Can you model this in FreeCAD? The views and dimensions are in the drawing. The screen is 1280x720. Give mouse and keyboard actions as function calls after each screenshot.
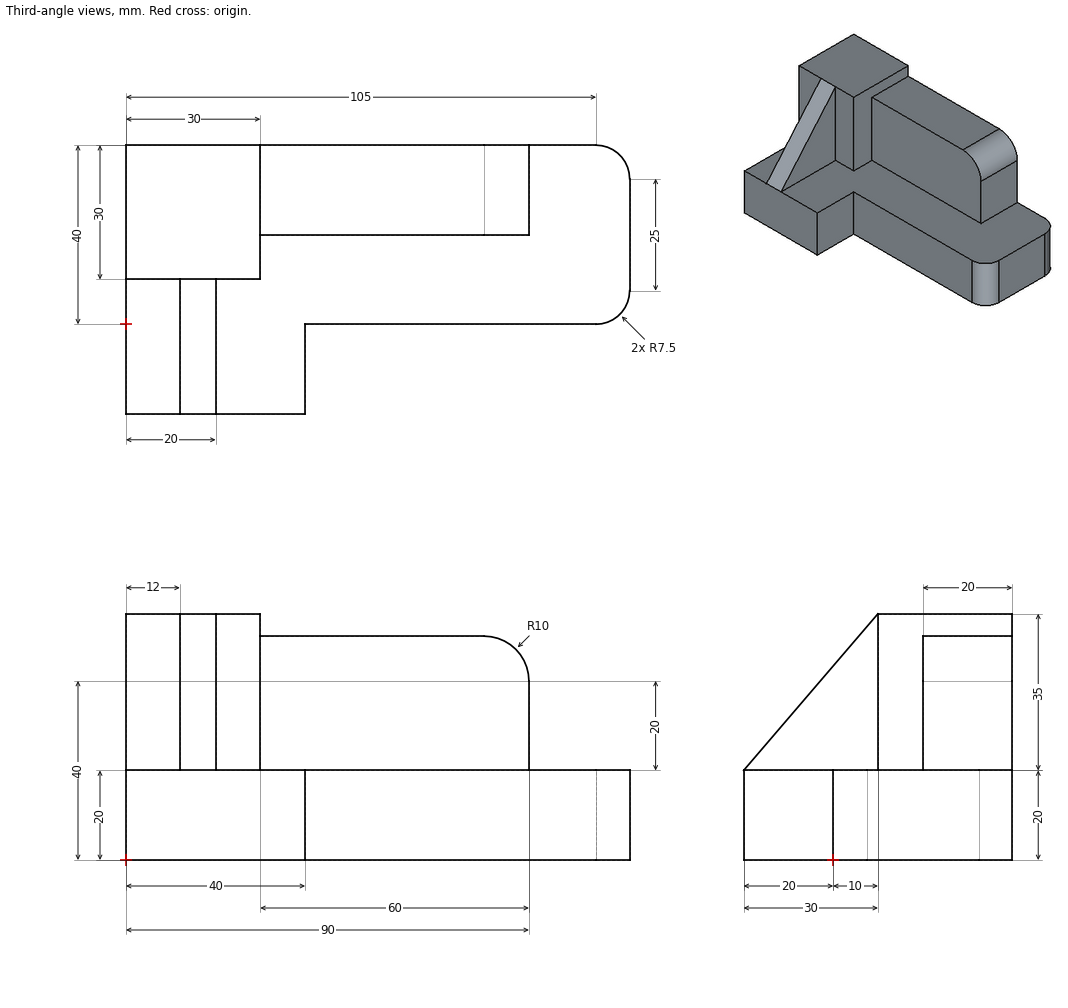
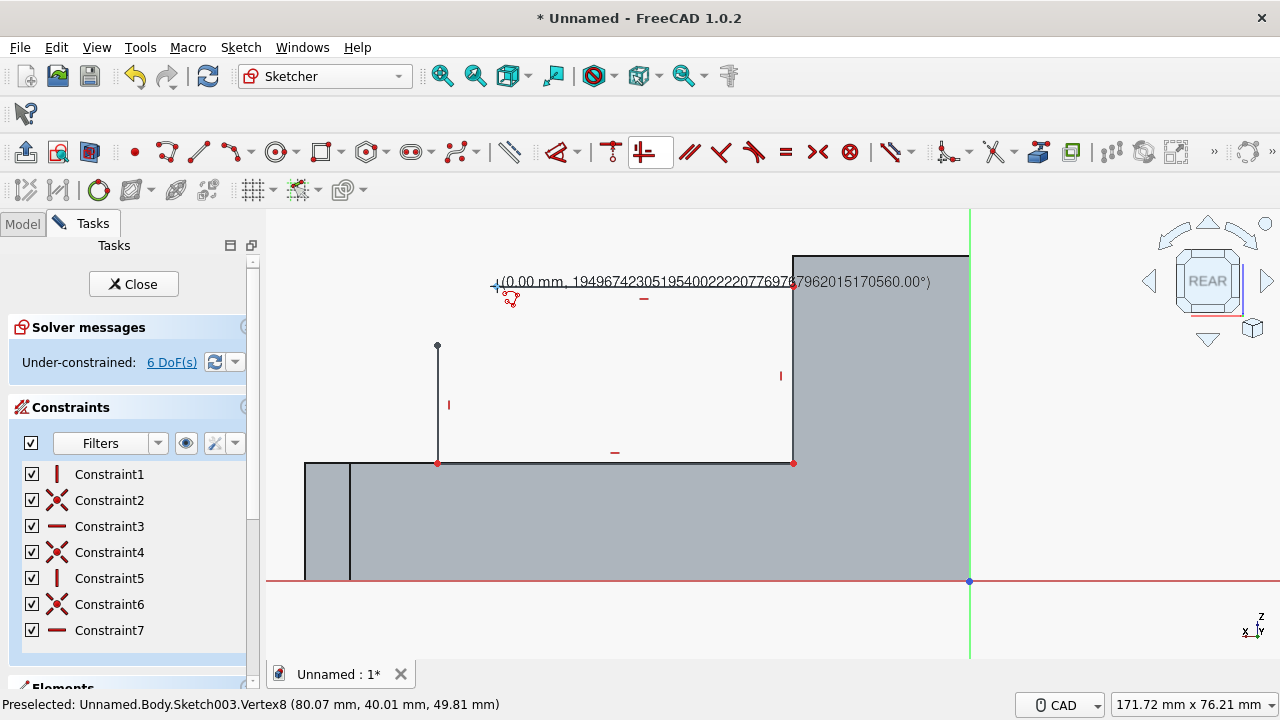
click(232, 152)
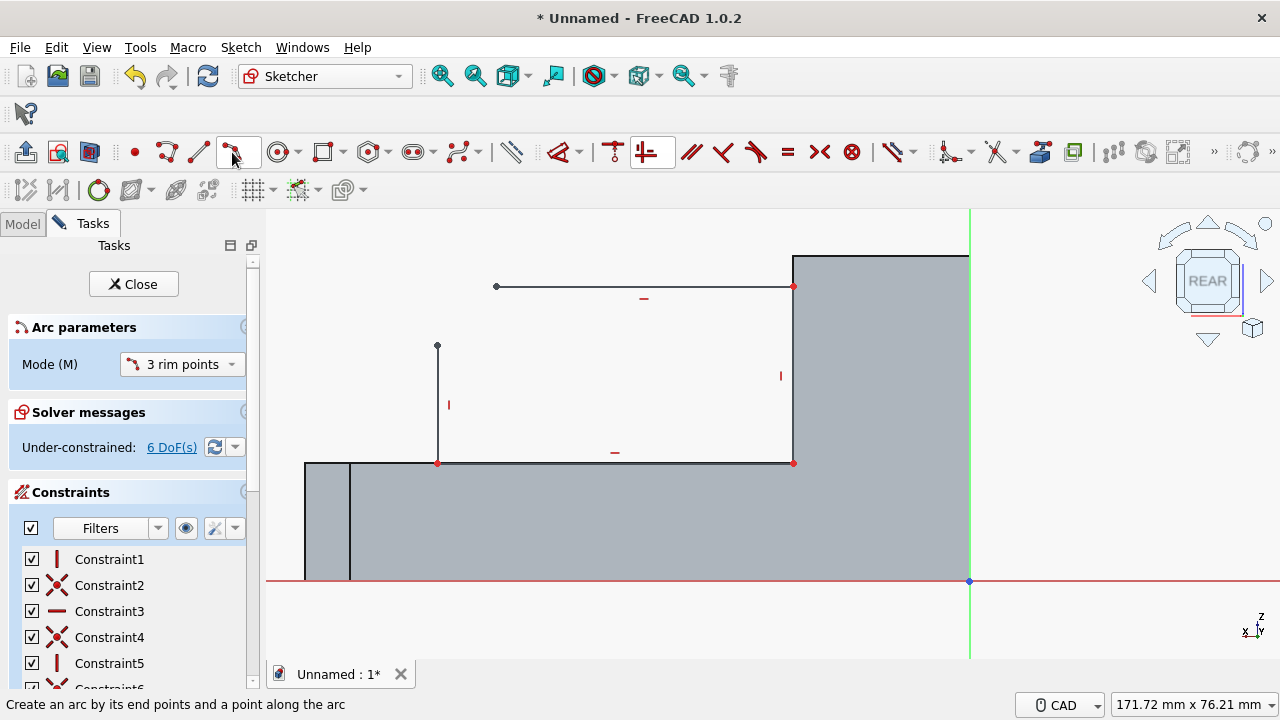
click(497, 287)
click(438, 346)
click(456, 303)
key(Escape)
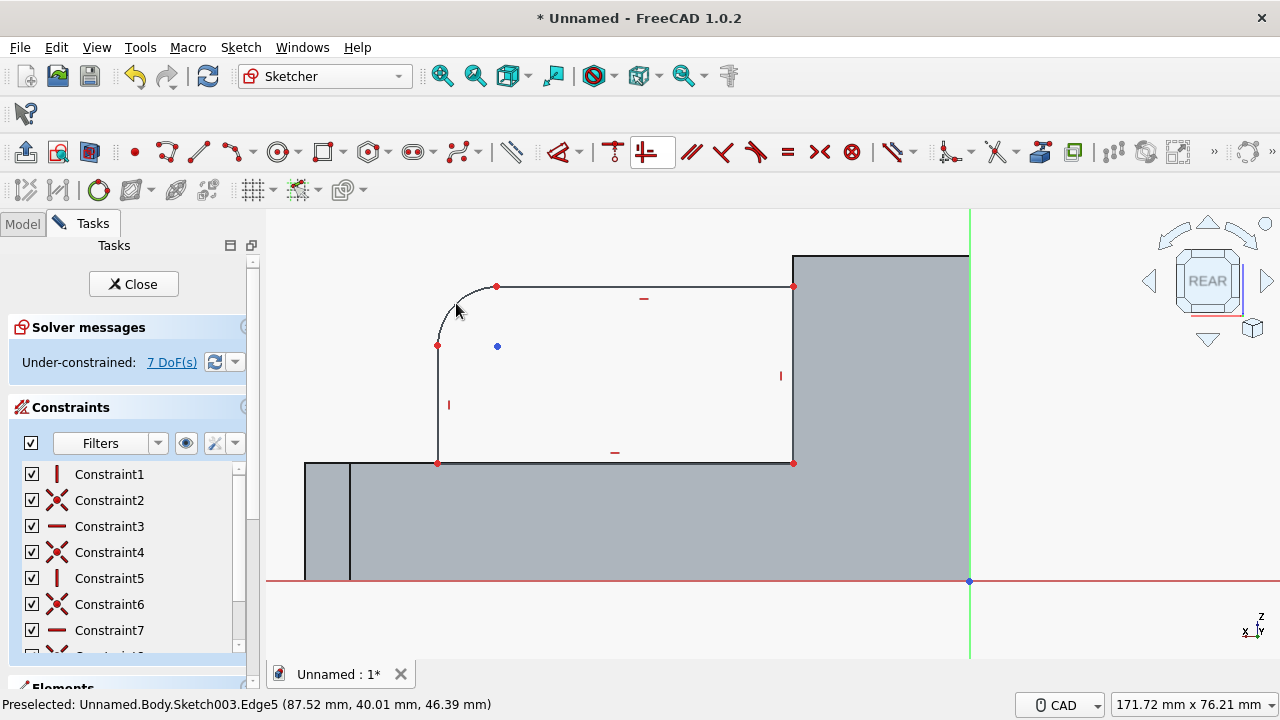
click(438, 381)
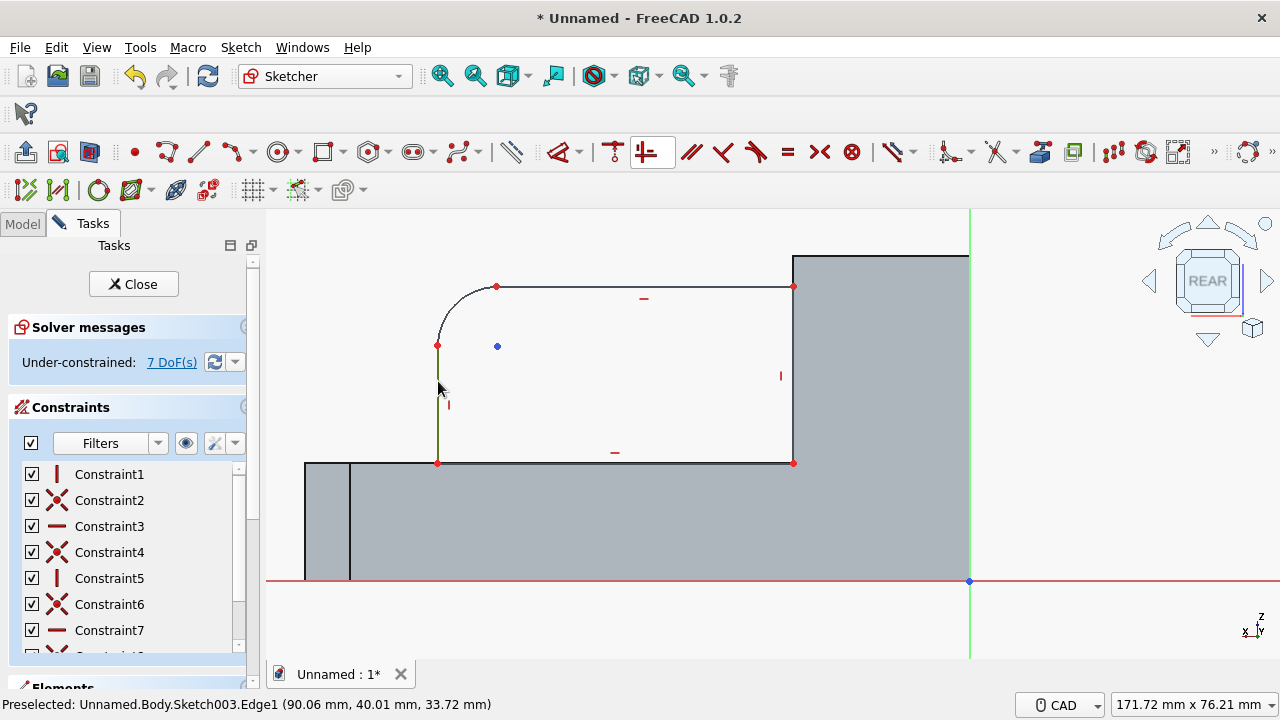
click(470, 294)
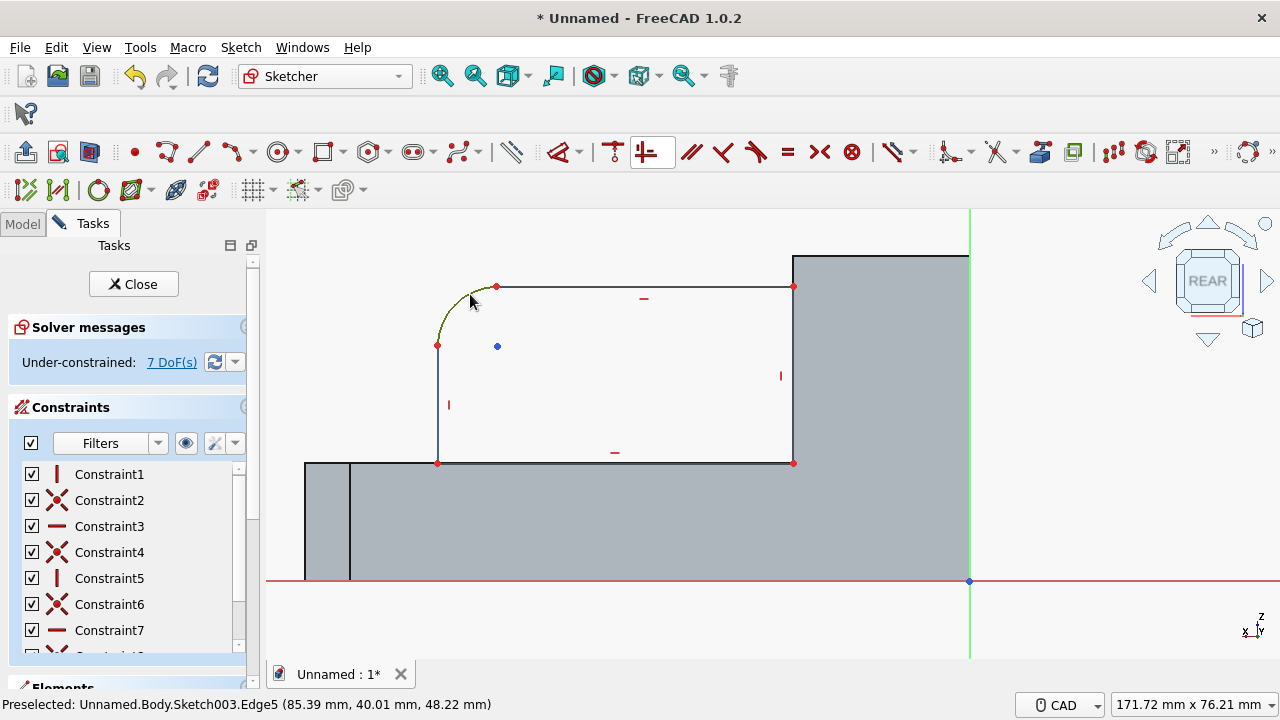
key(t)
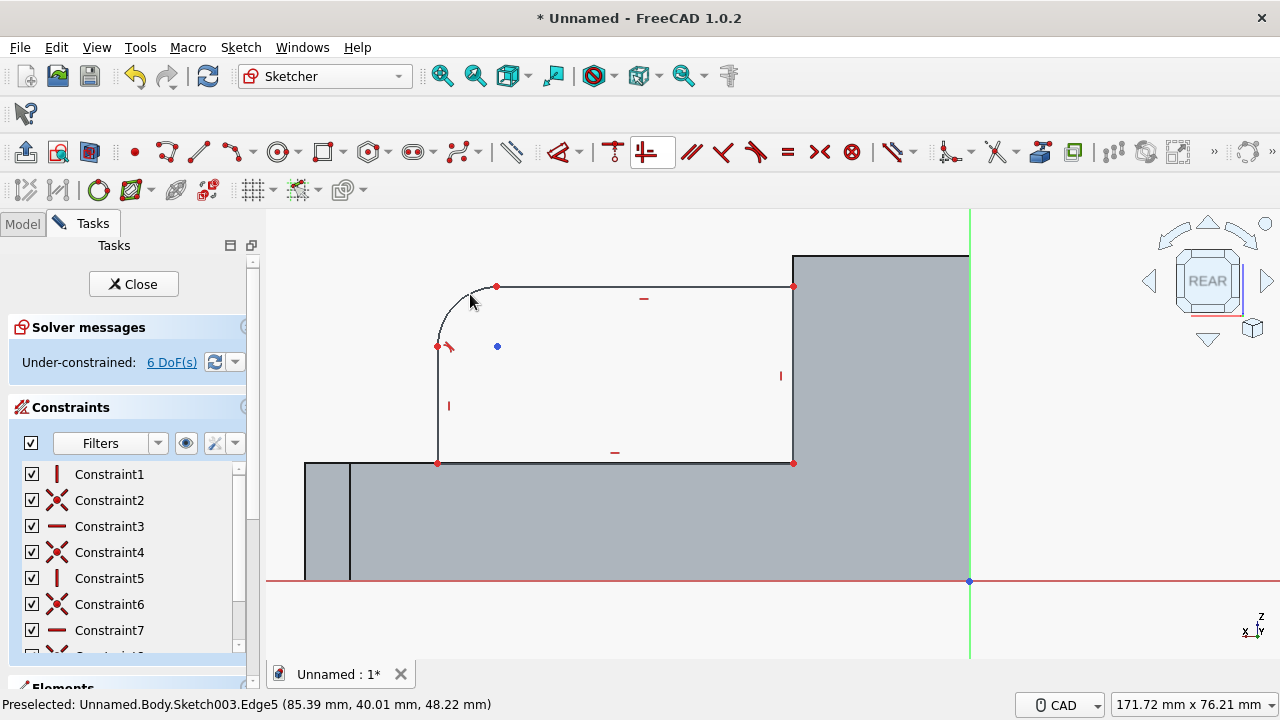
click(704, 287)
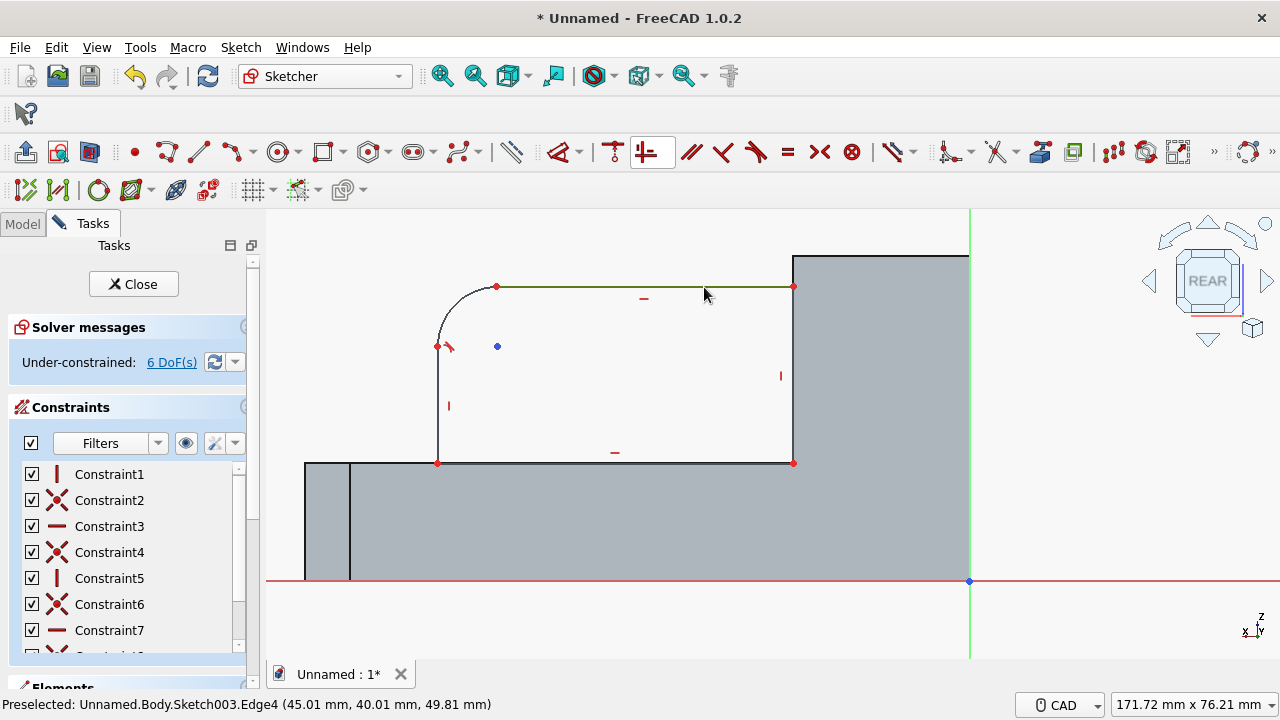
click(470, 294)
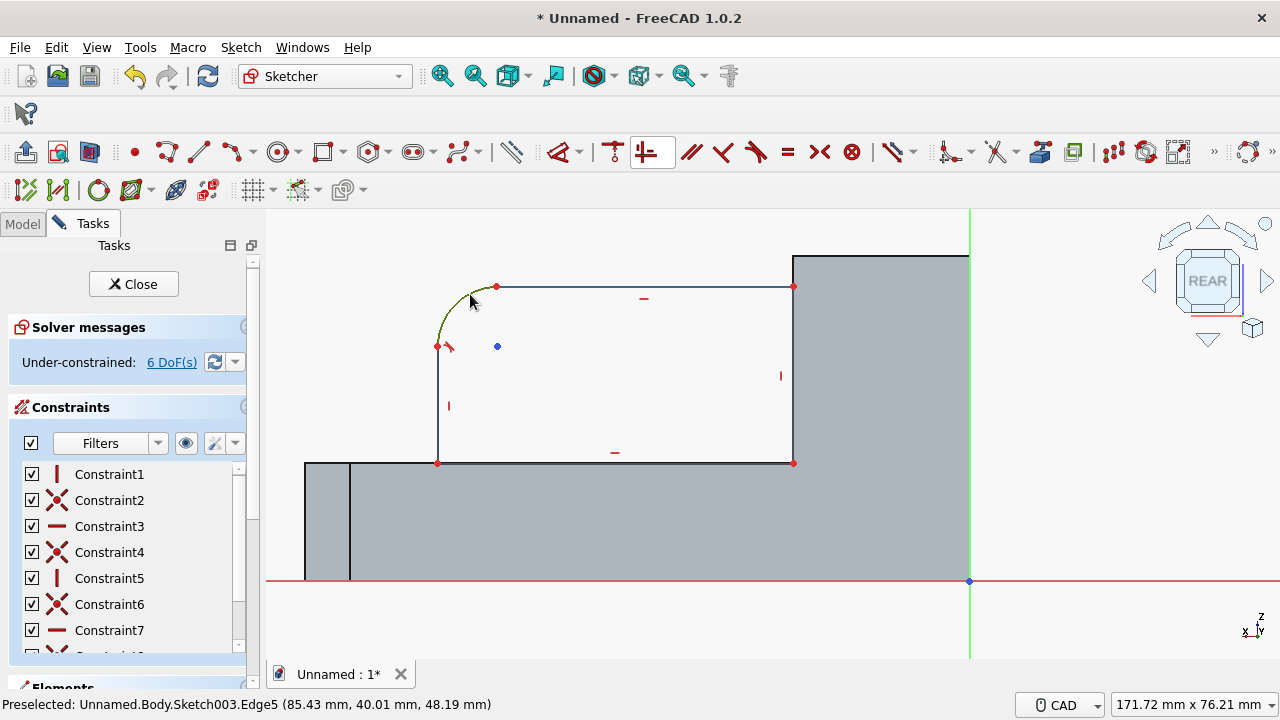
key(t)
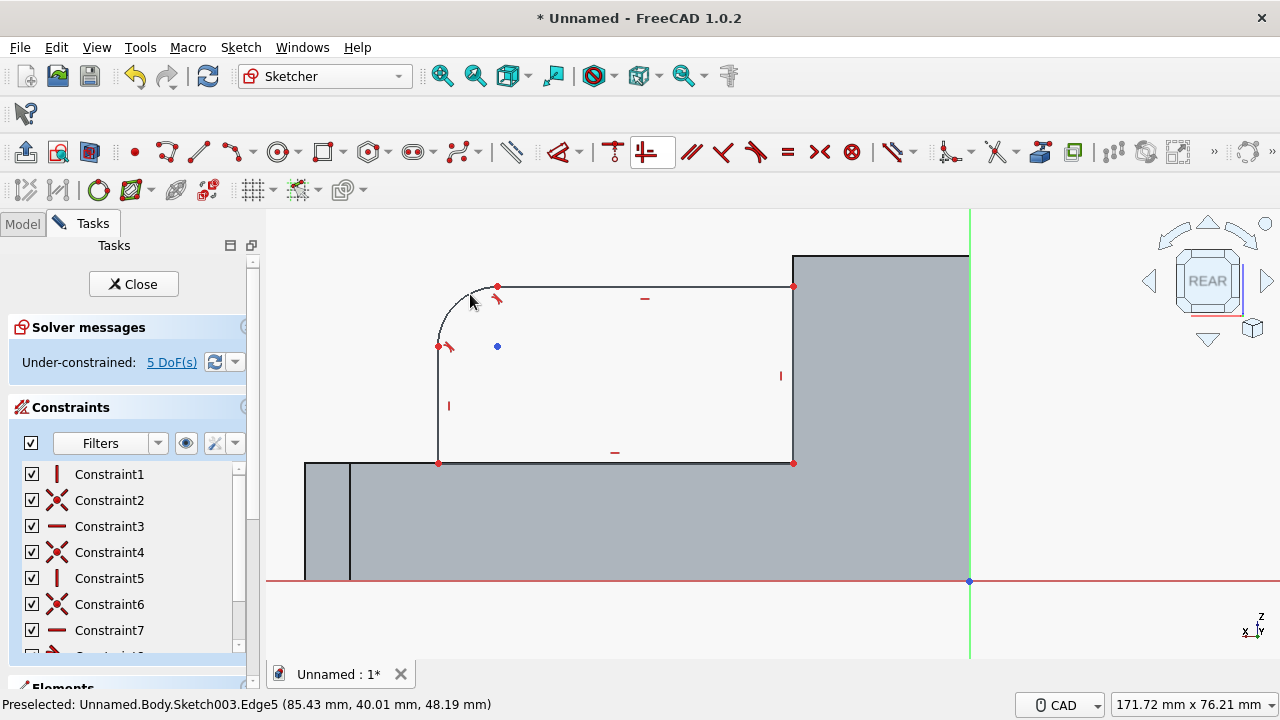
key(d)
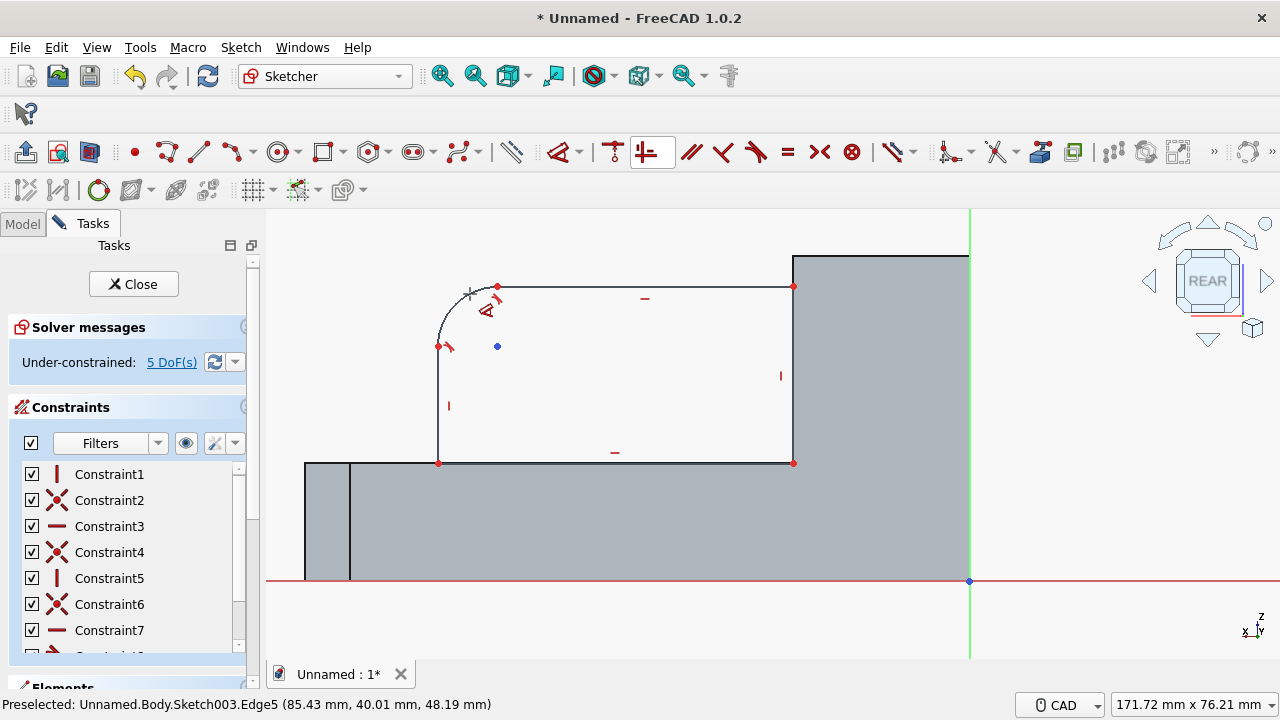
click(471, 294)
click(457, 265)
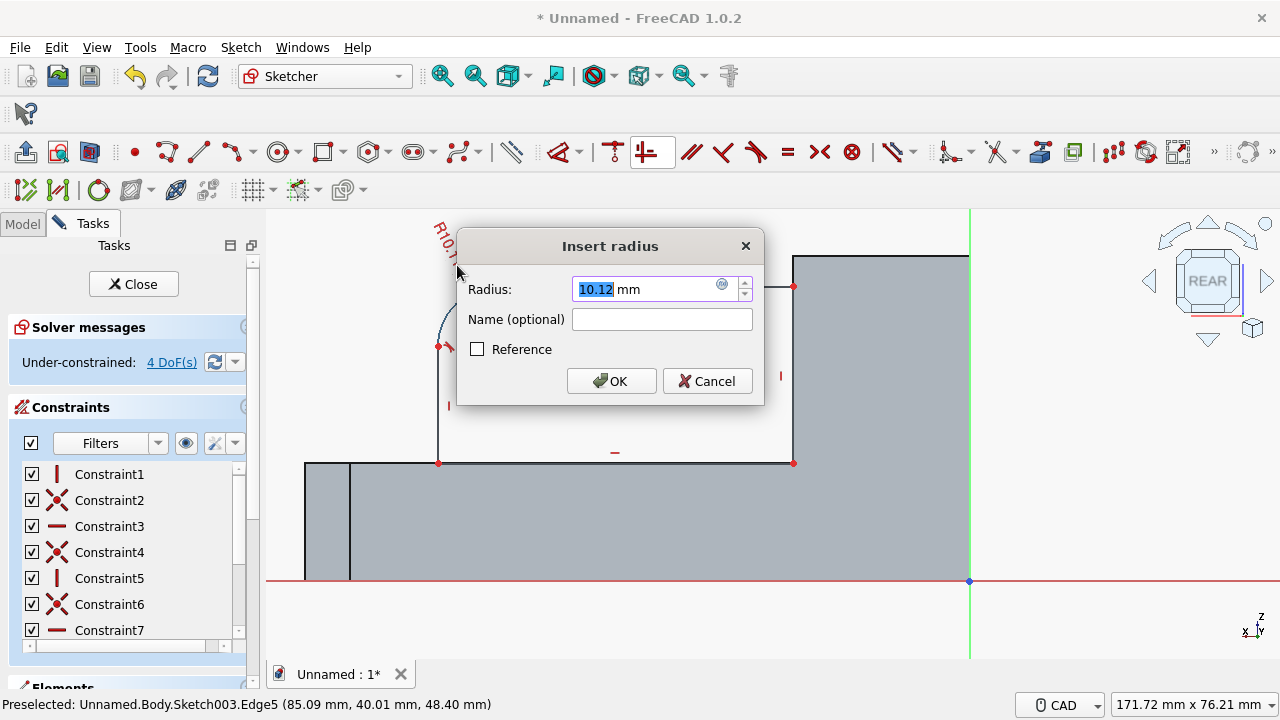
text(10)
key(Return)